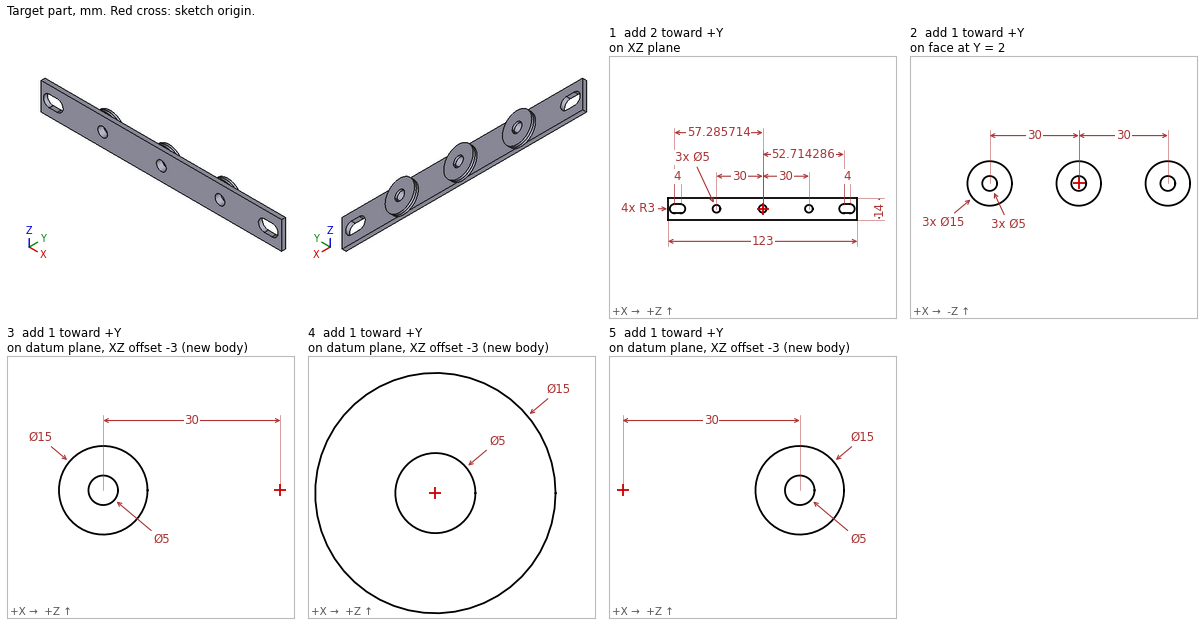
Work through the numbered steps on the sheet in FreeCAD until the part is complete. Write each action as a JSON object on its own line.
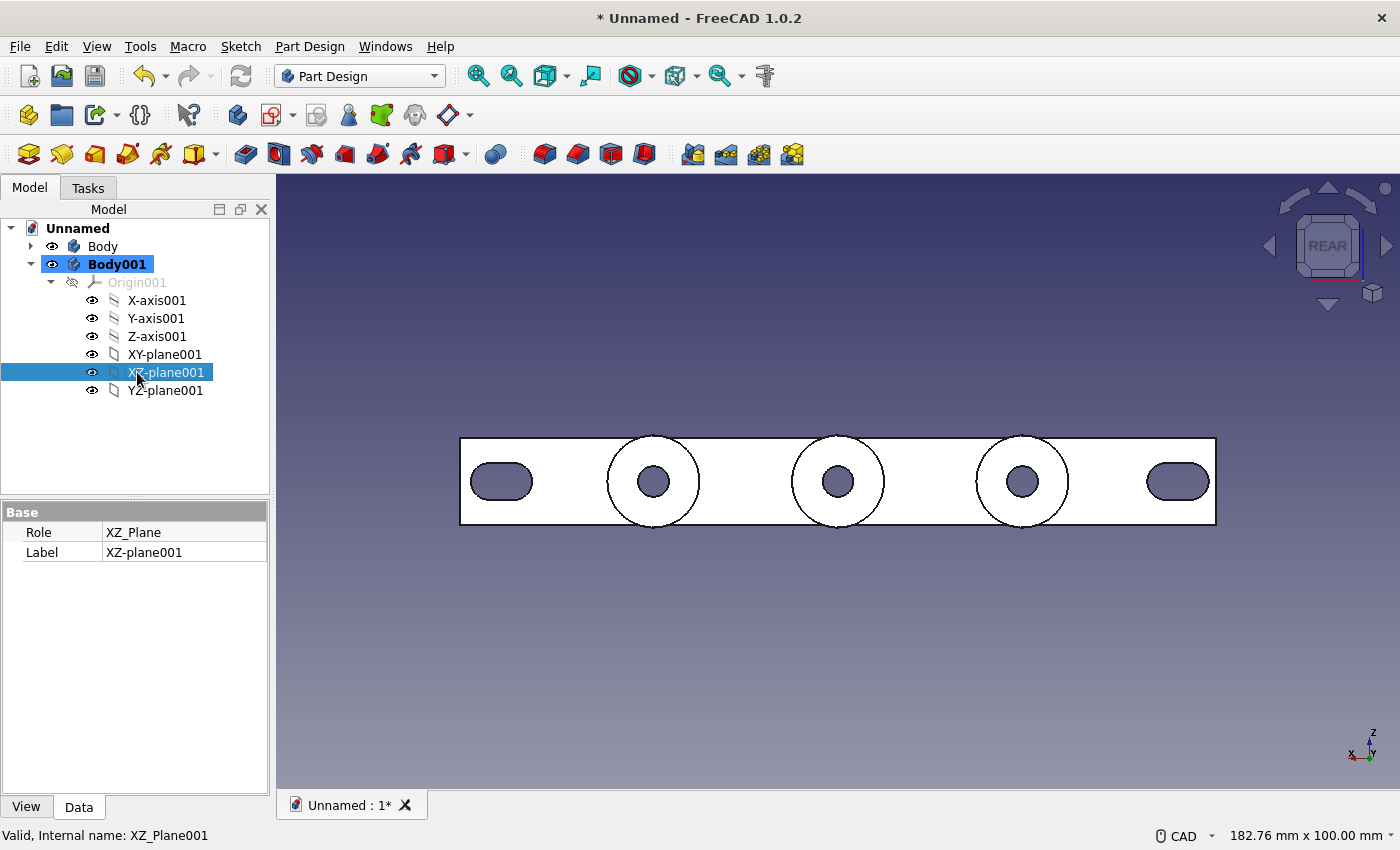
{"action": "left_click", "coordinate": [448, 116]}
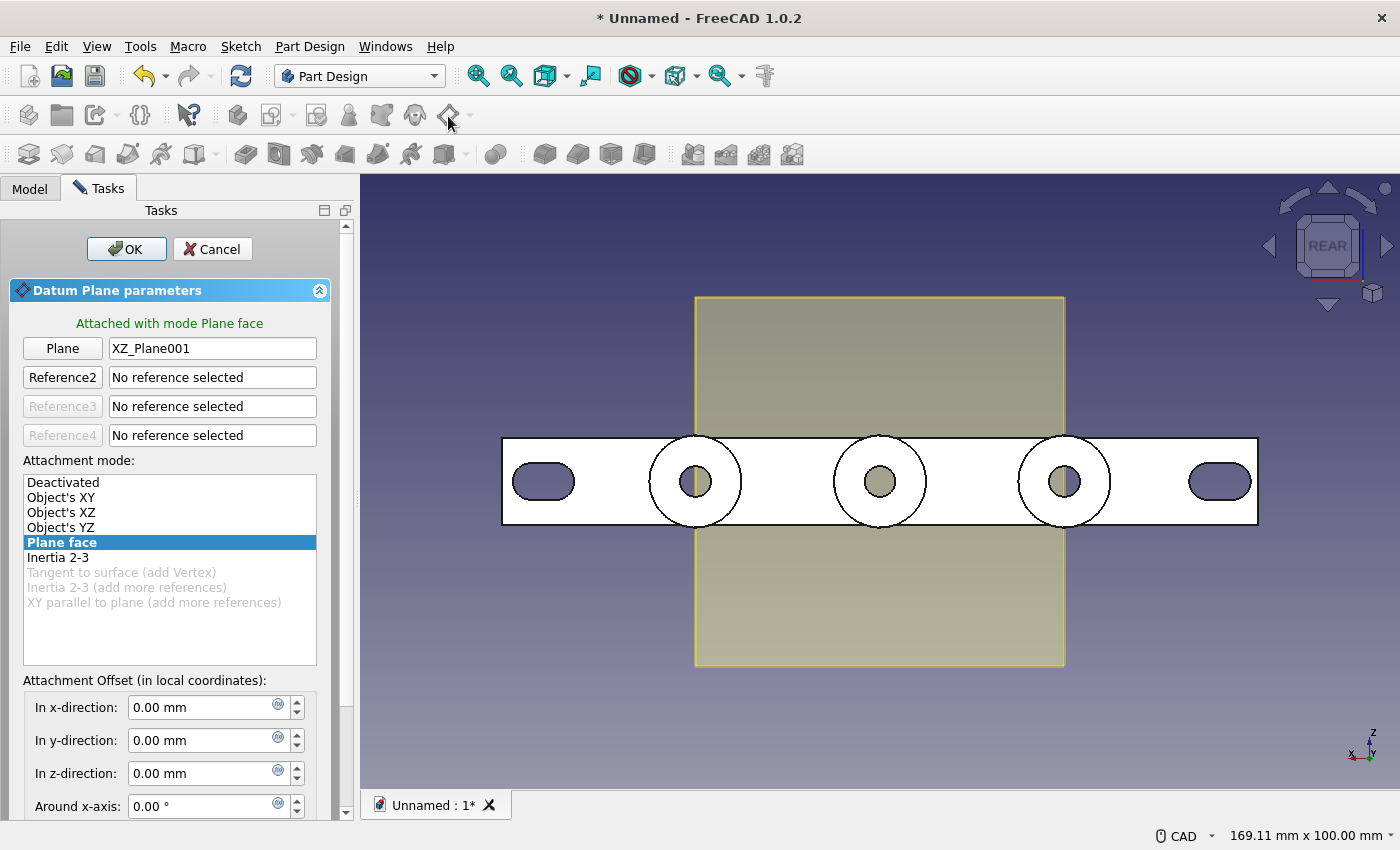
{"action": "triple_click", "coordinate": [210, 774]}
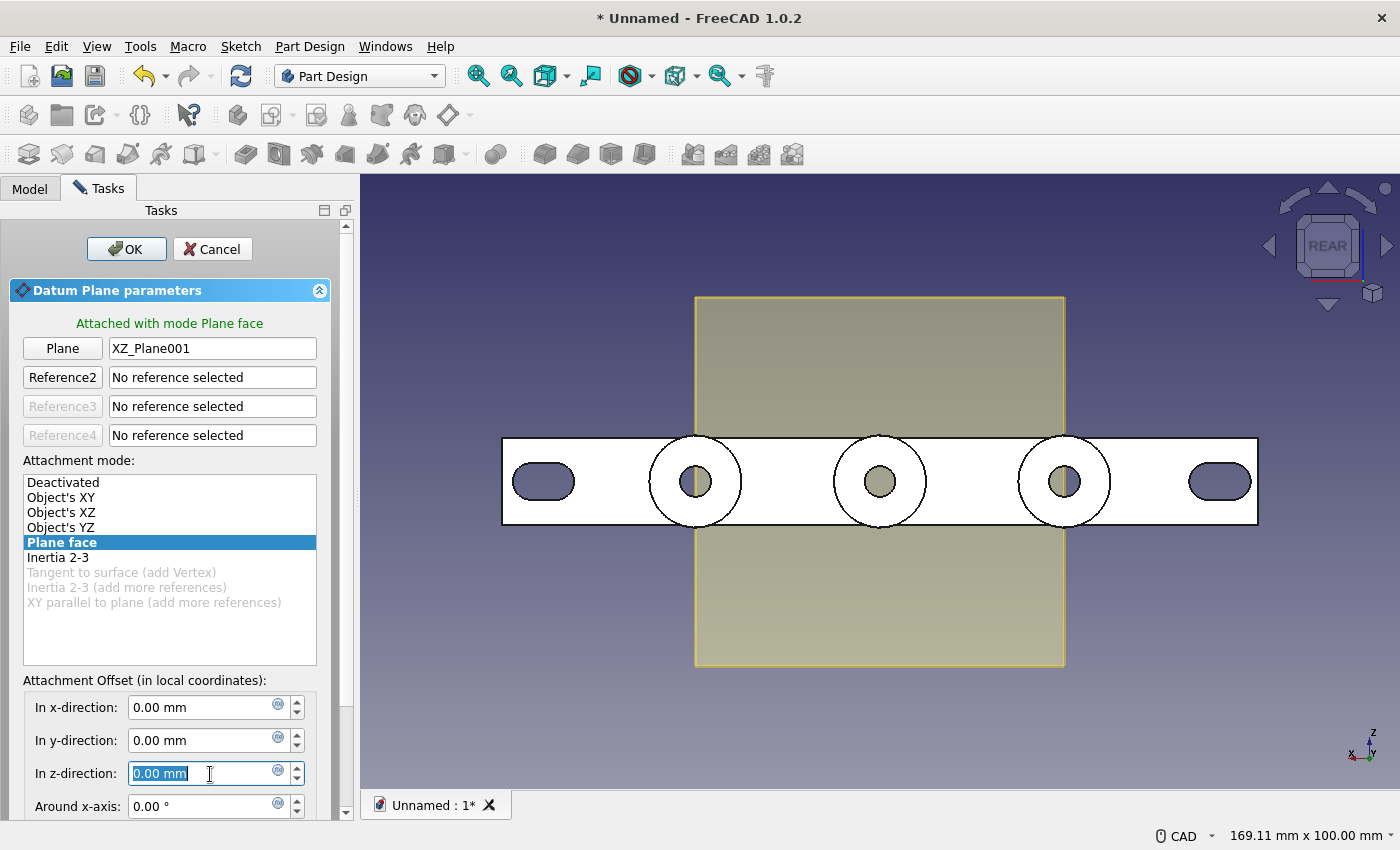
{"action": "type", "text": "-3"}
{"action": "key", "text": "Tab"}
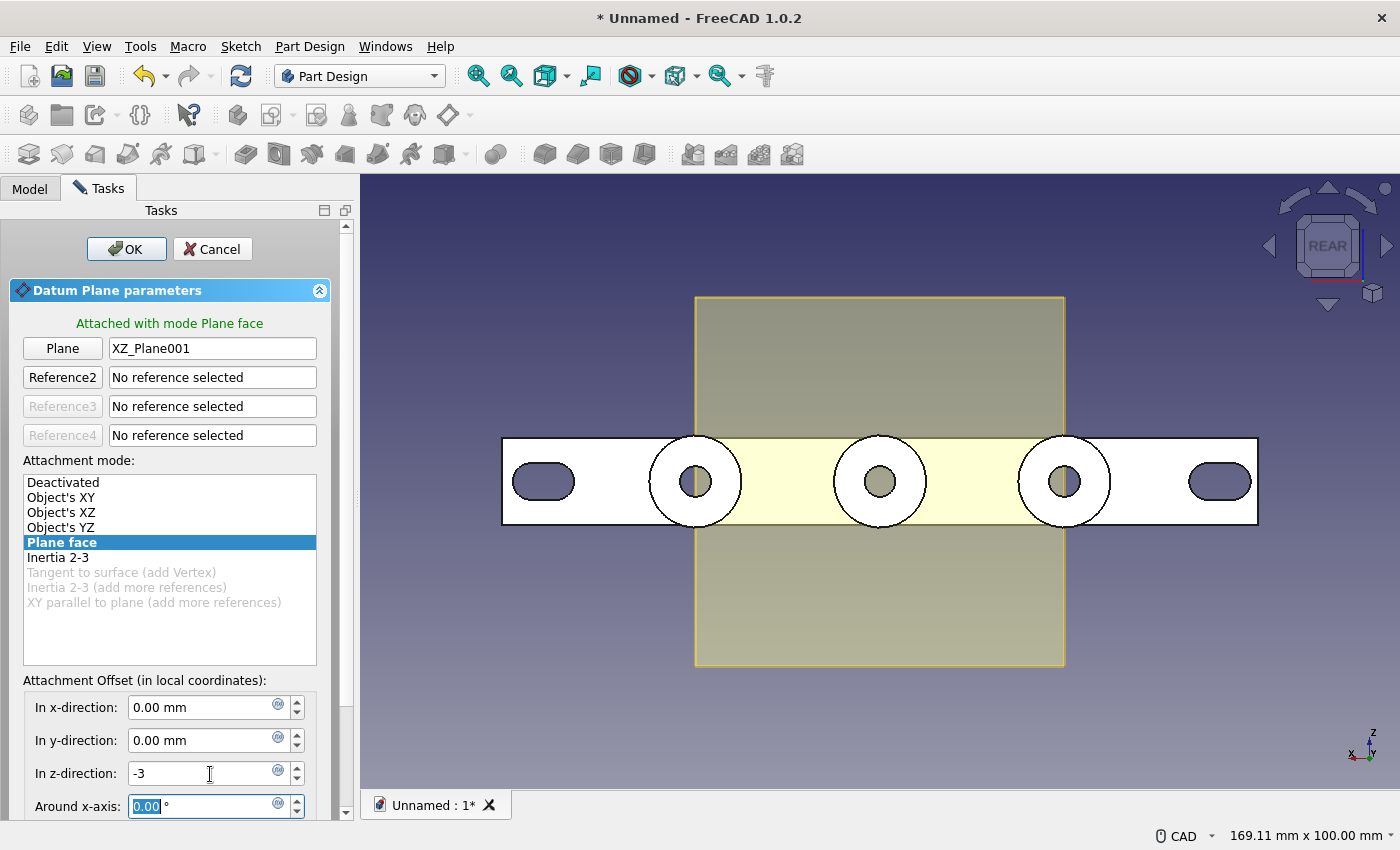
{"action": "left_click", "coordinate": [127, 249]}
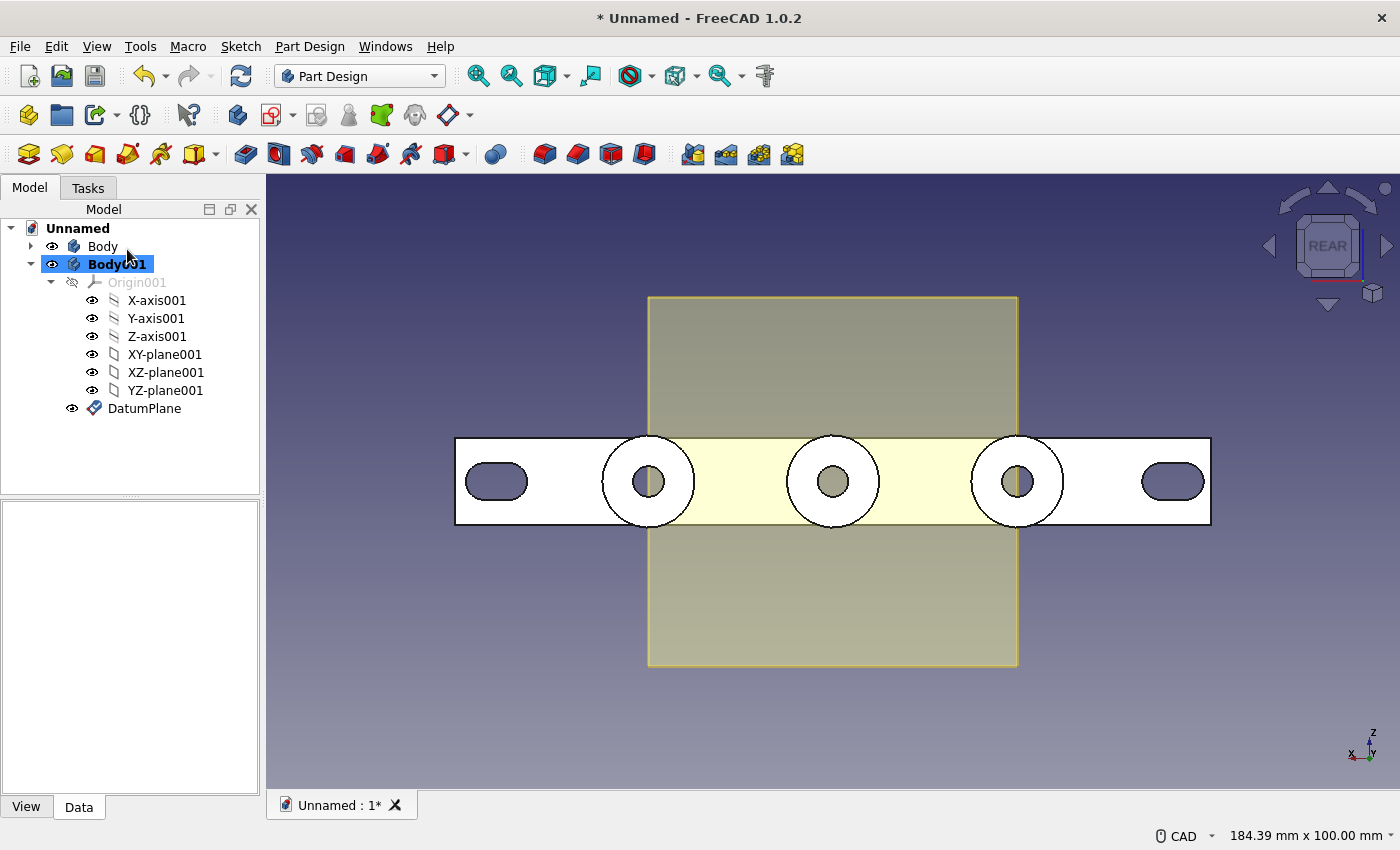
{"action": "left_click", "coordinate": [117, 408]}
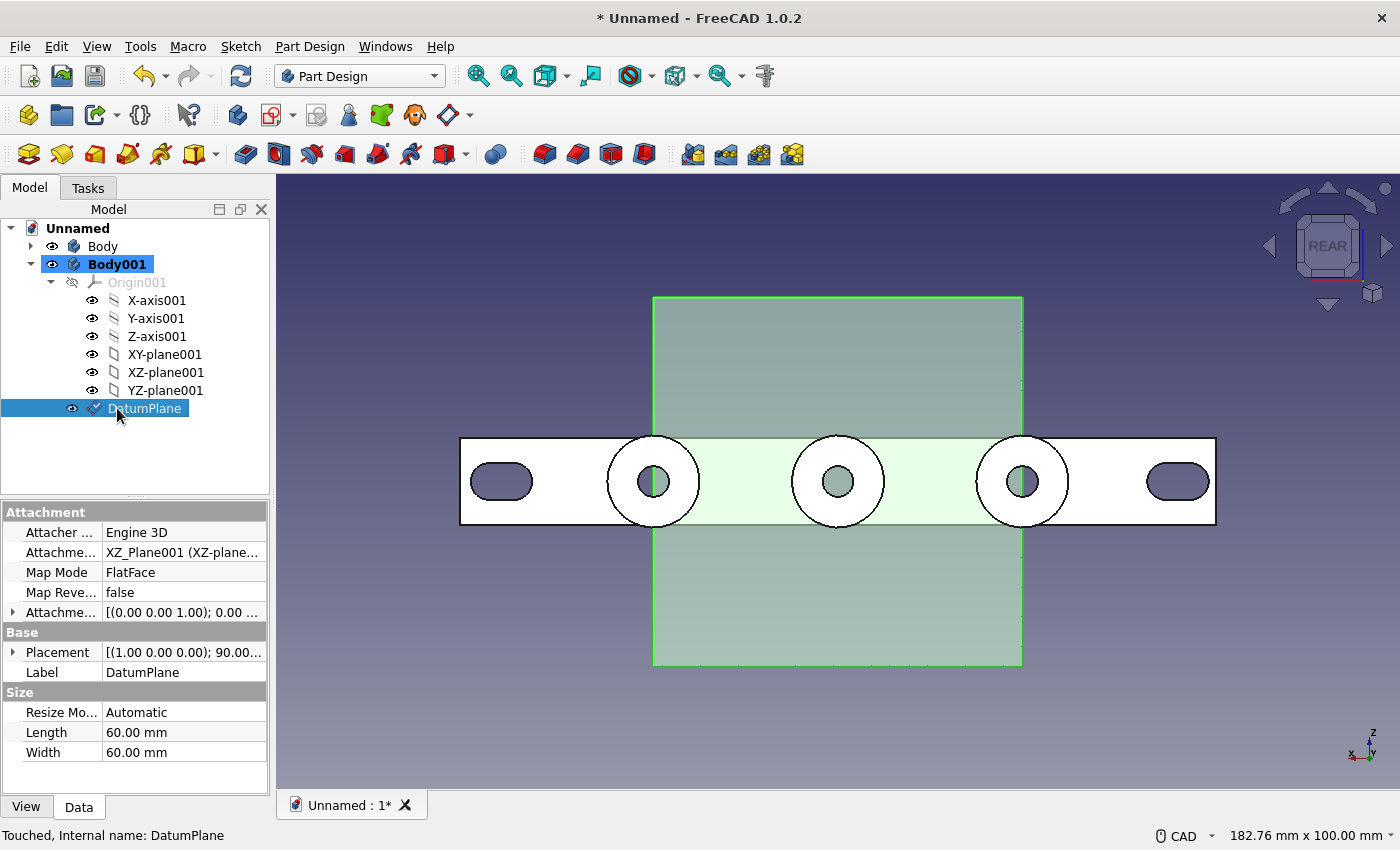
{"action": "left_click", "coordinate": [270, 116]}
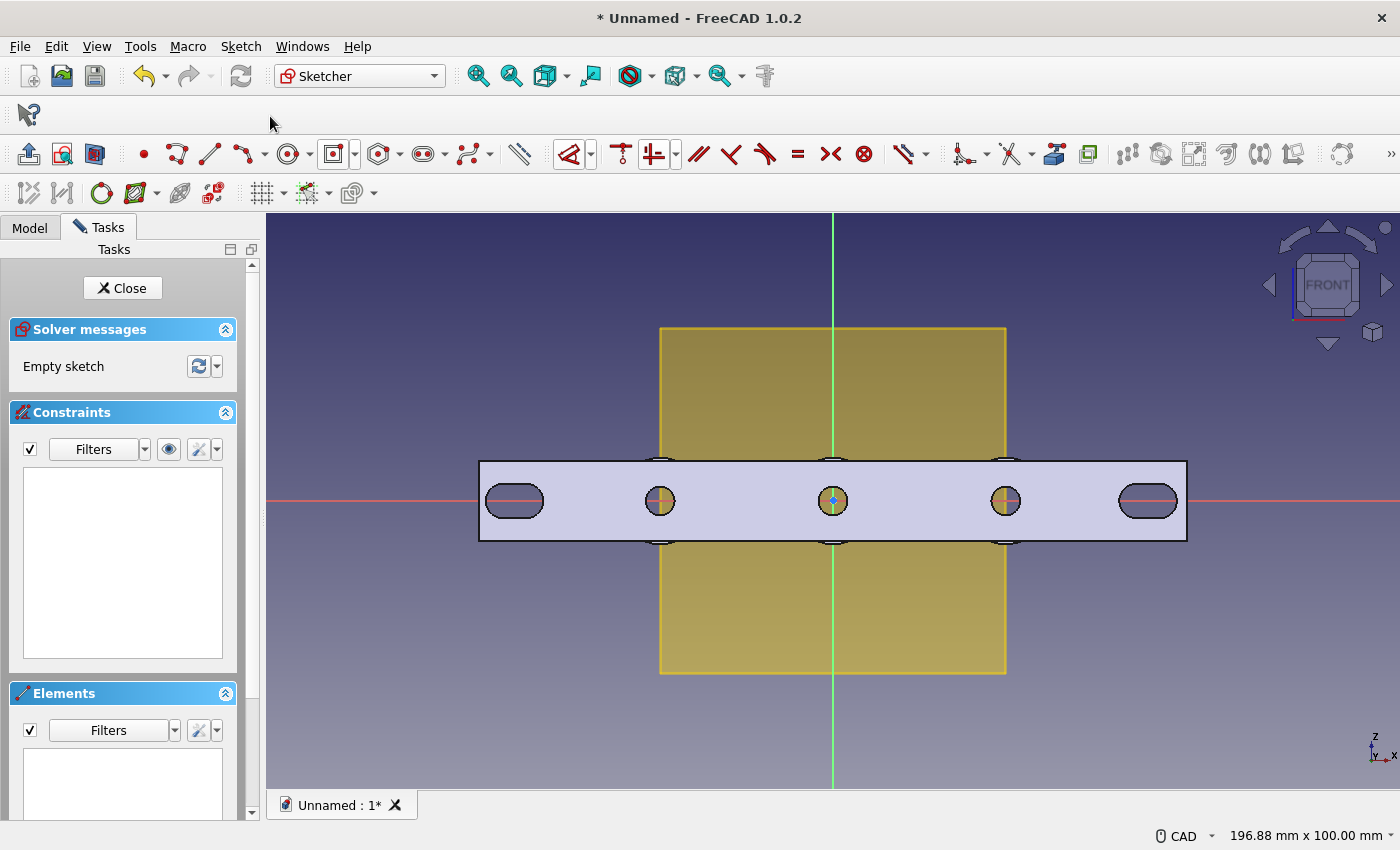
{"action": "scroll", "coordinate": [626, 501], "scroll_direction": "up", "scroll_amount": 7}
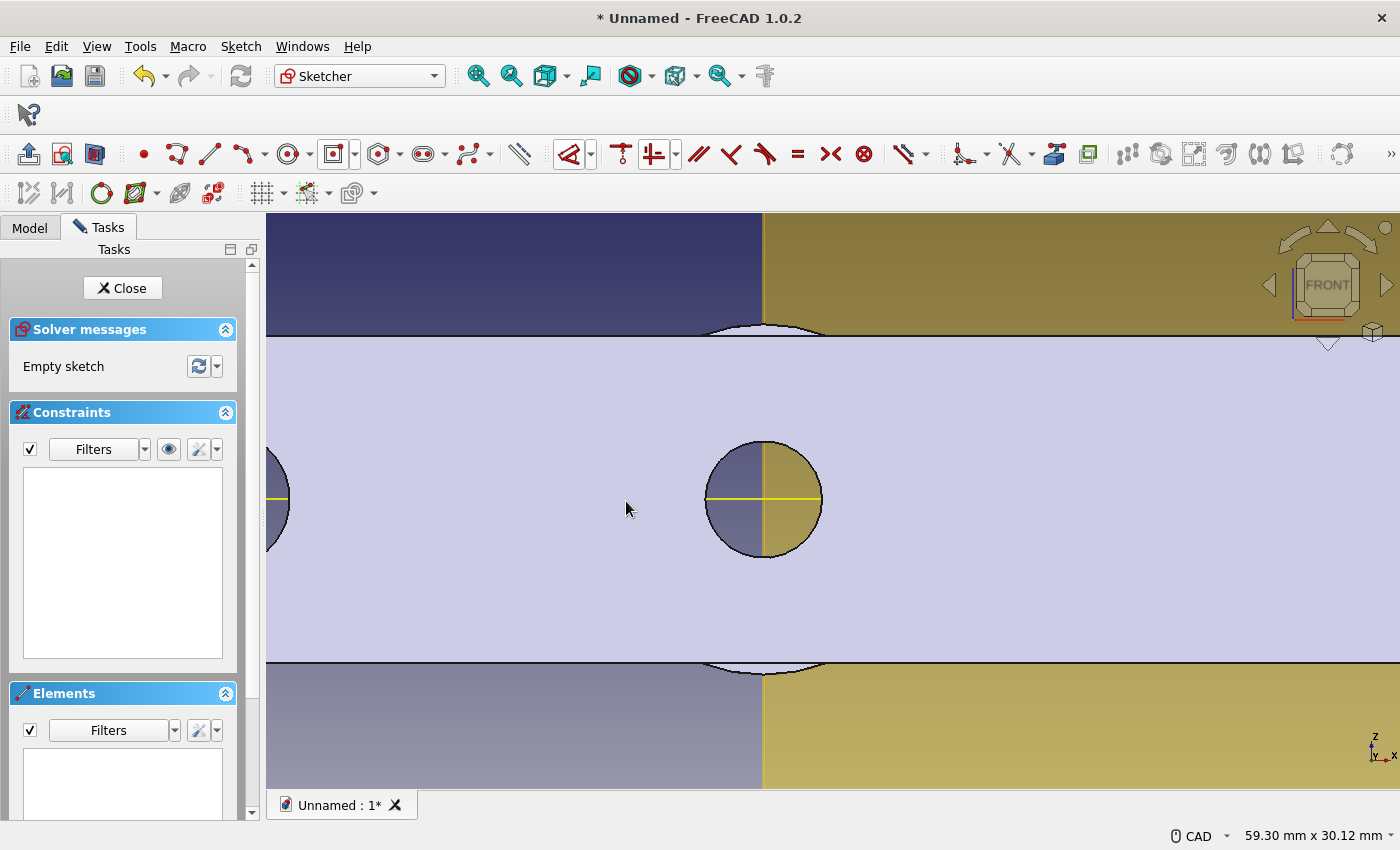
{"action": "left_click", "coordinate": [288, 154]}